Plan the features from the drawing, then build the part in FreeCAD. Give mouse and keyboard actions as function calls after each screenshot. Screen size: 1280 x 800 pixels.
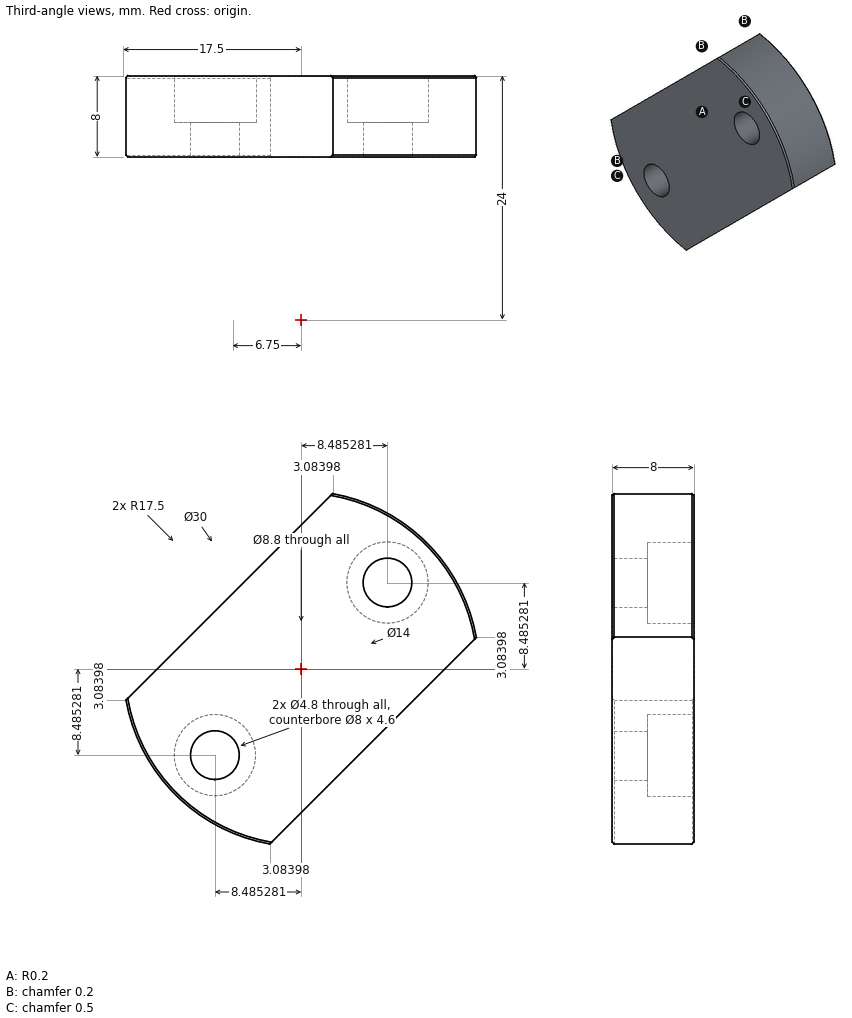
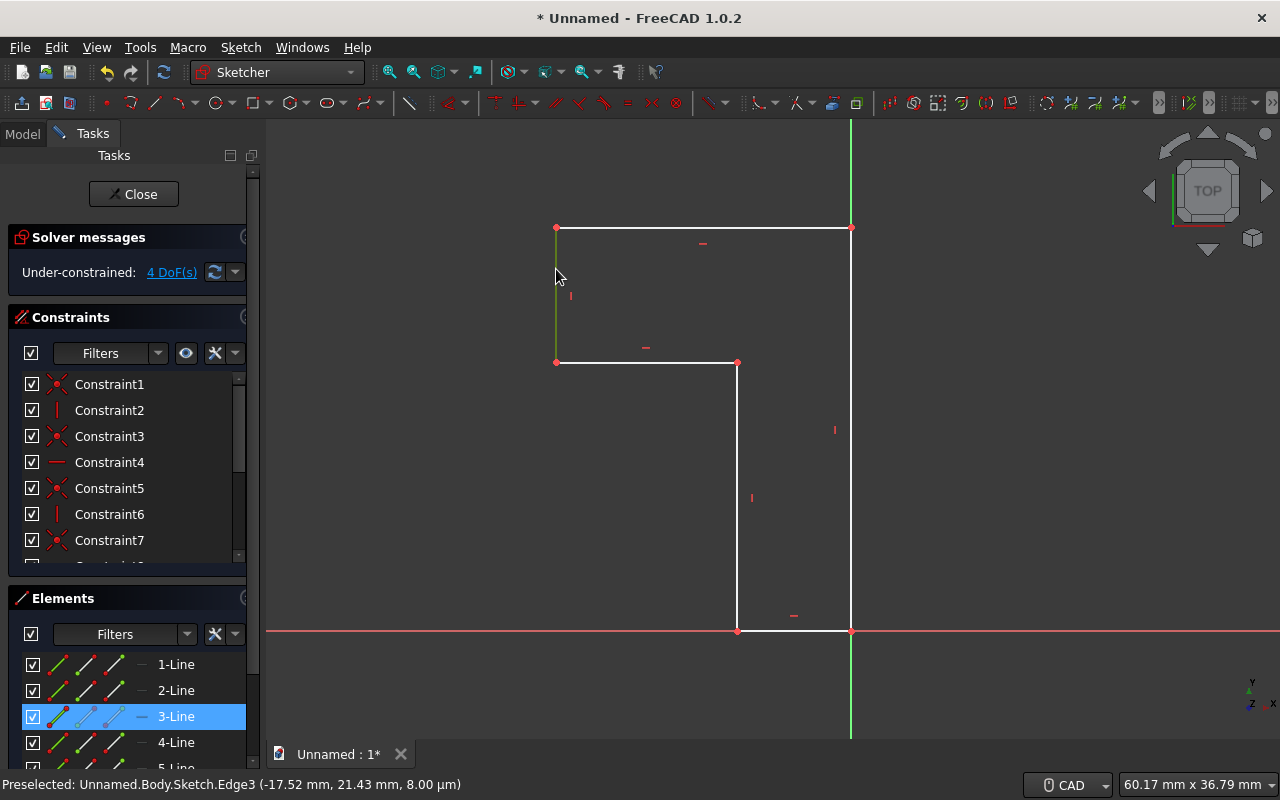
key(i)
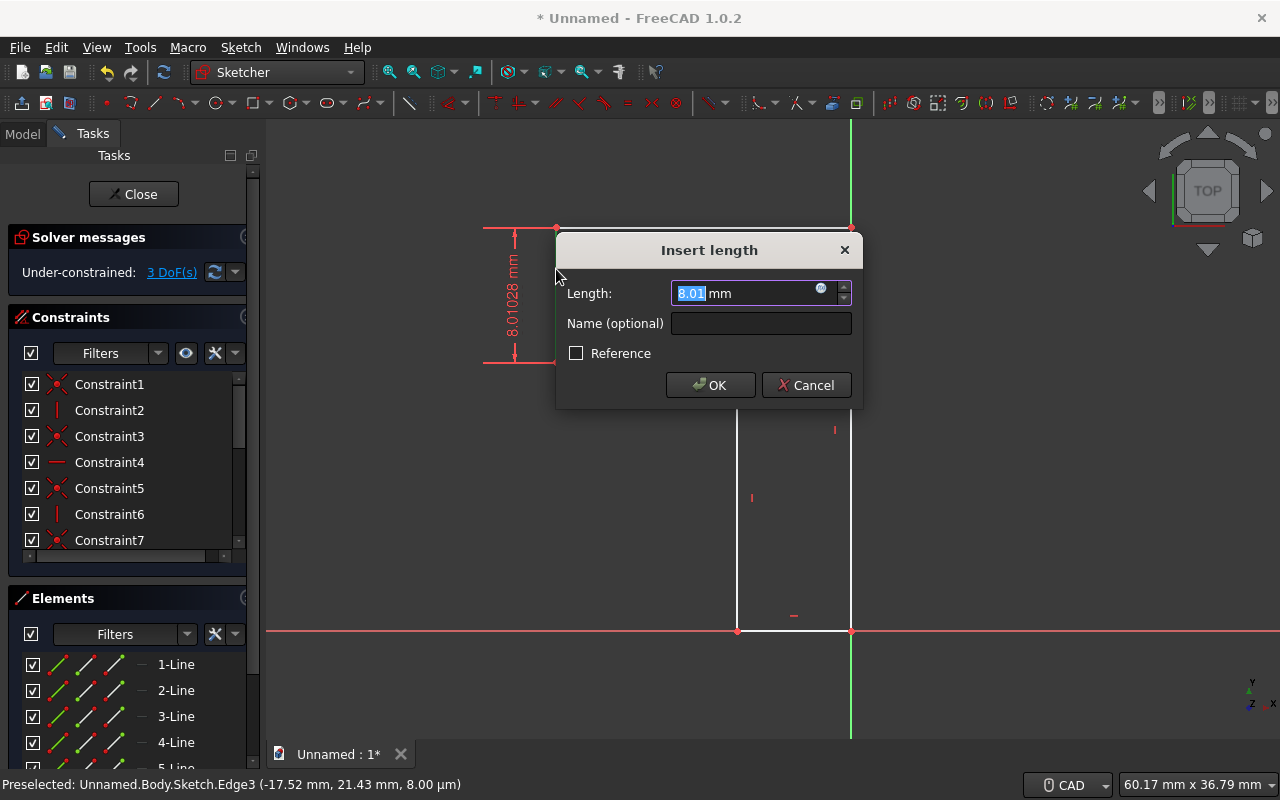
text(8)
key(Return)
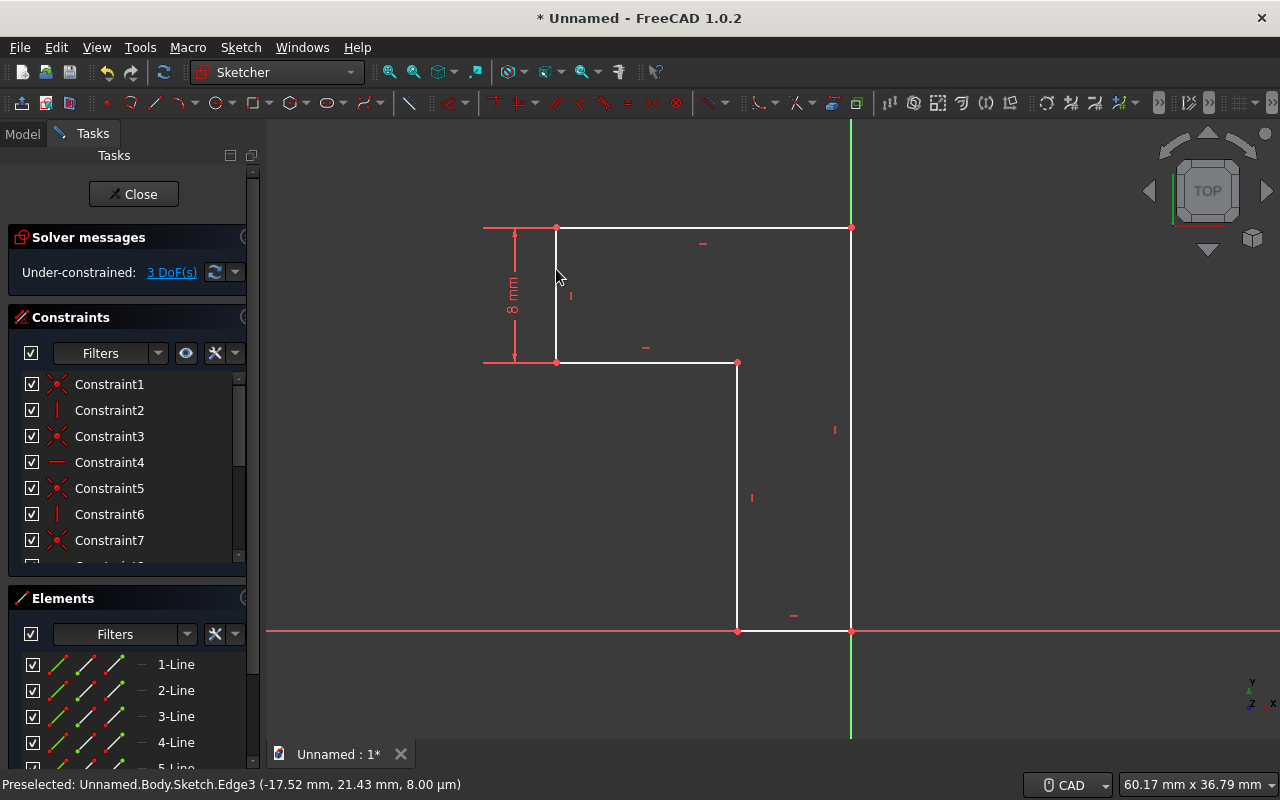
click(851, 510)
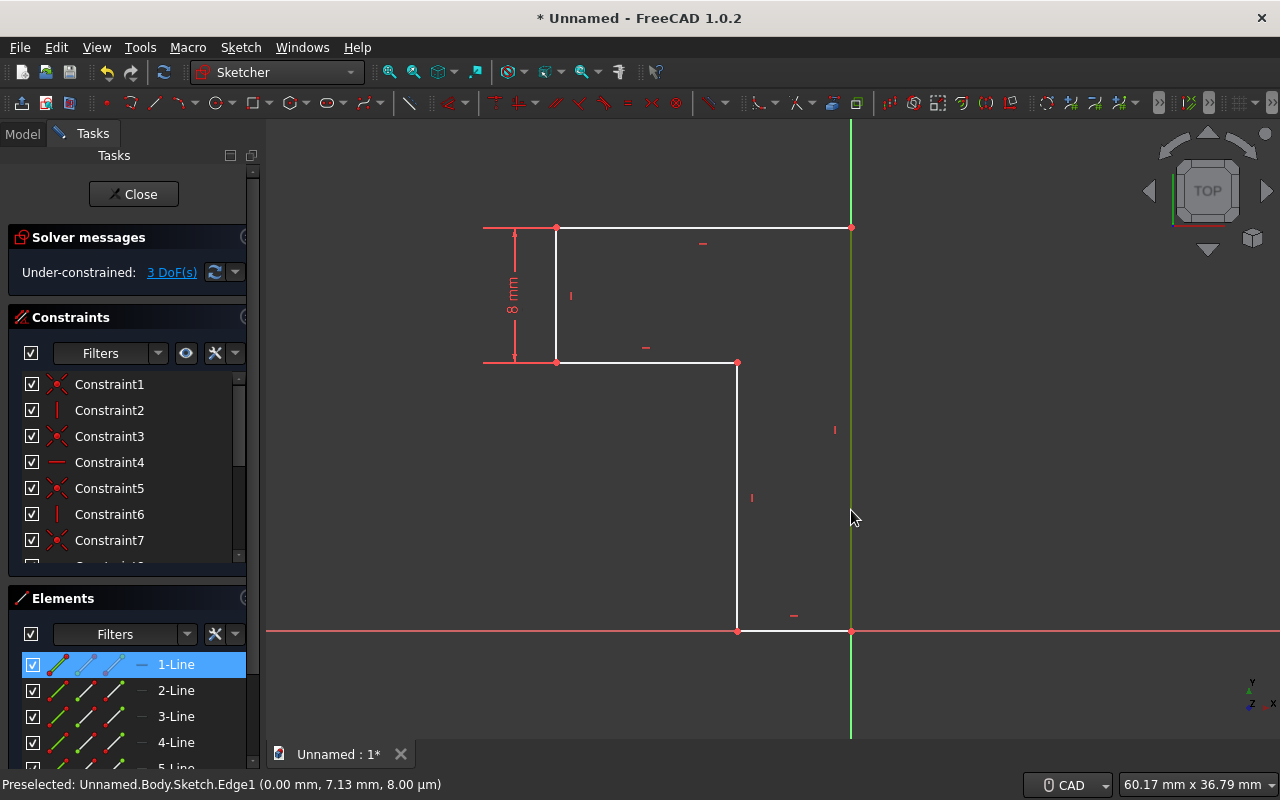
click(468, 104)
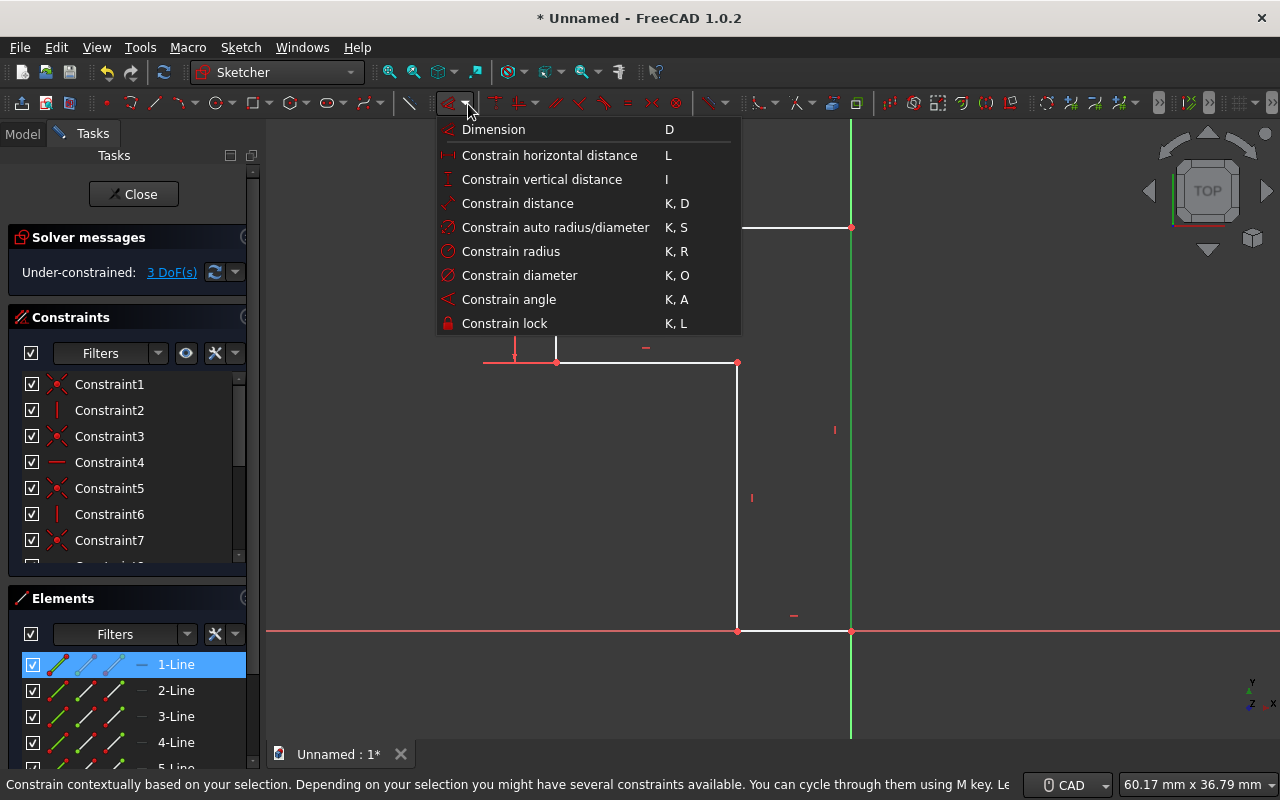
click(589, 179)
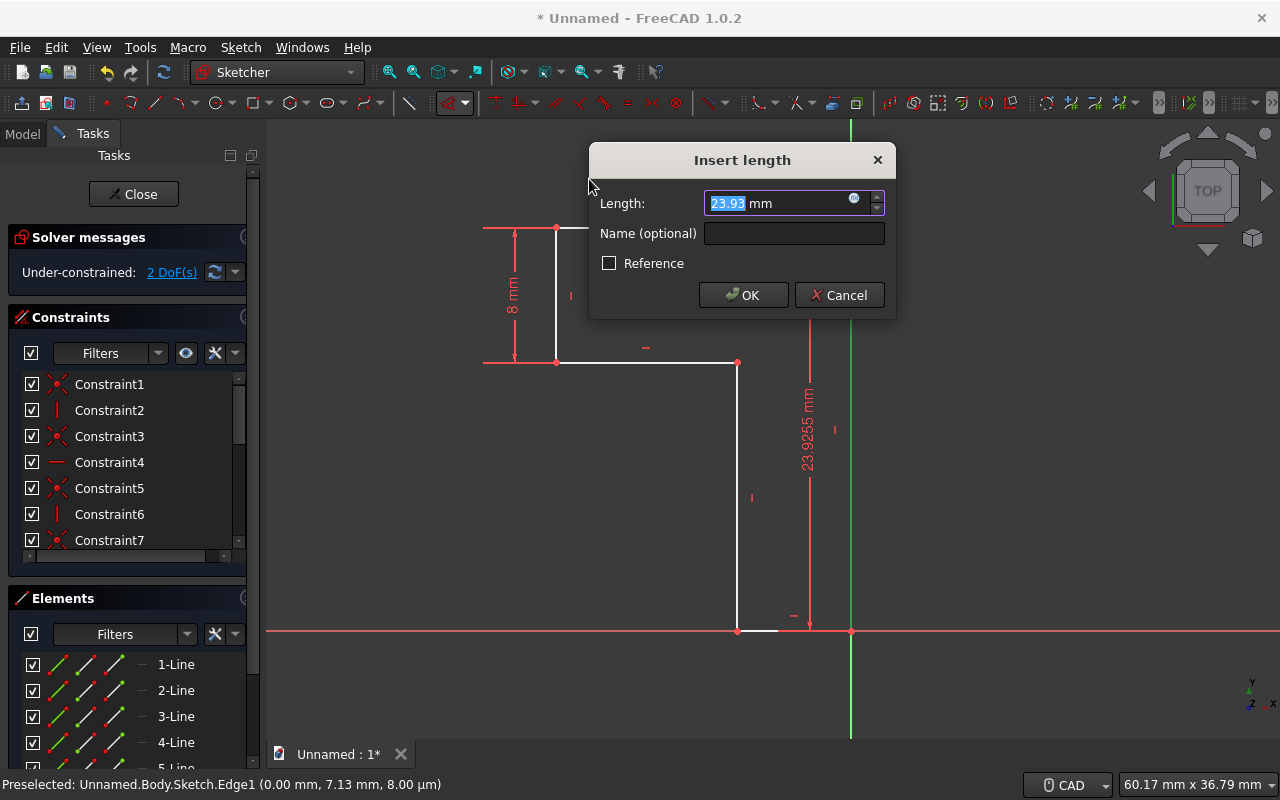
text(24)
key(Return)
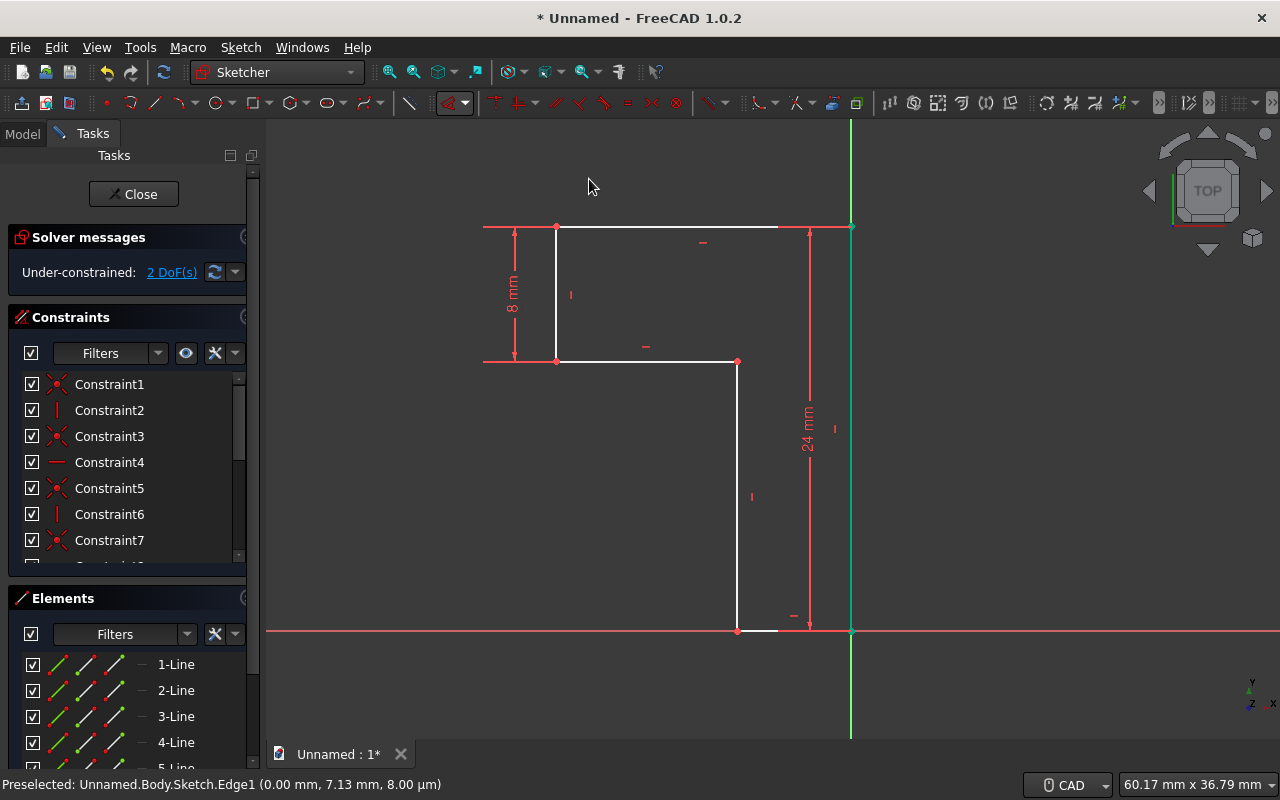
click(763, 227)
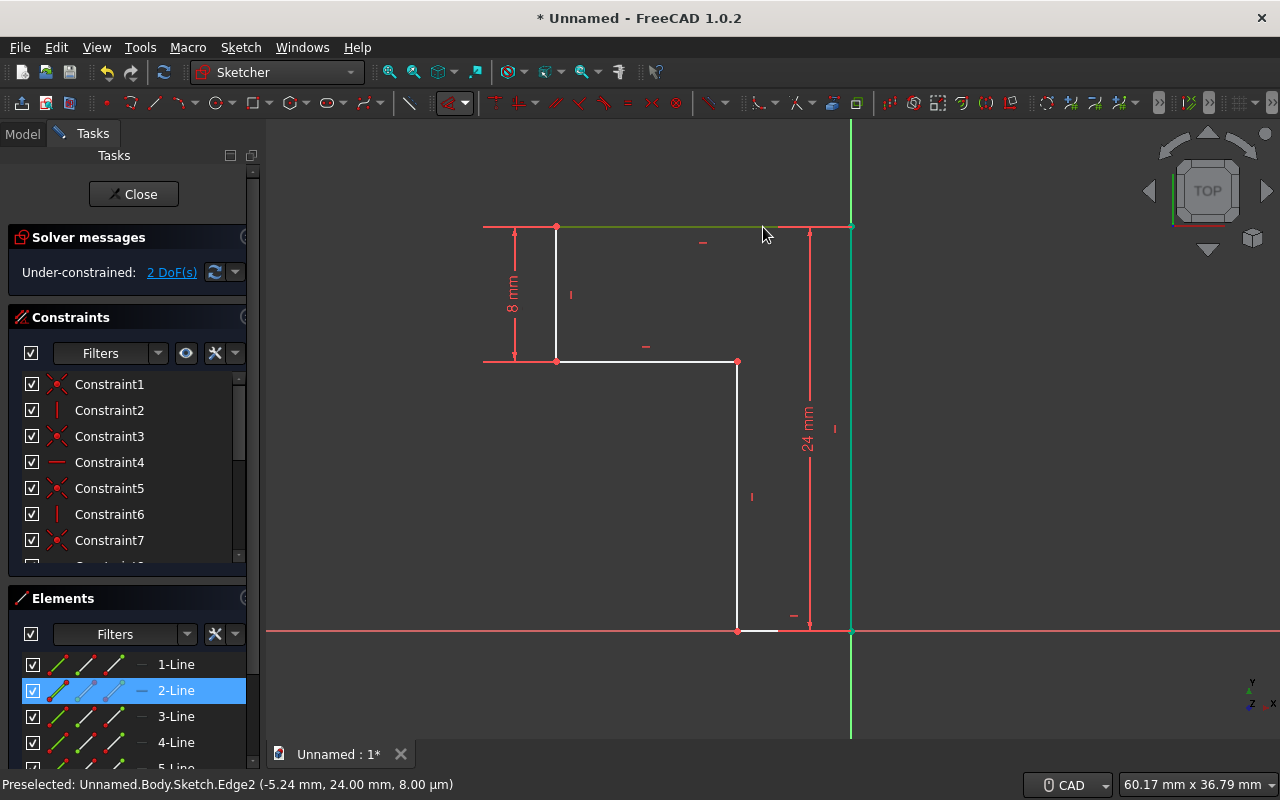
click(468, 104)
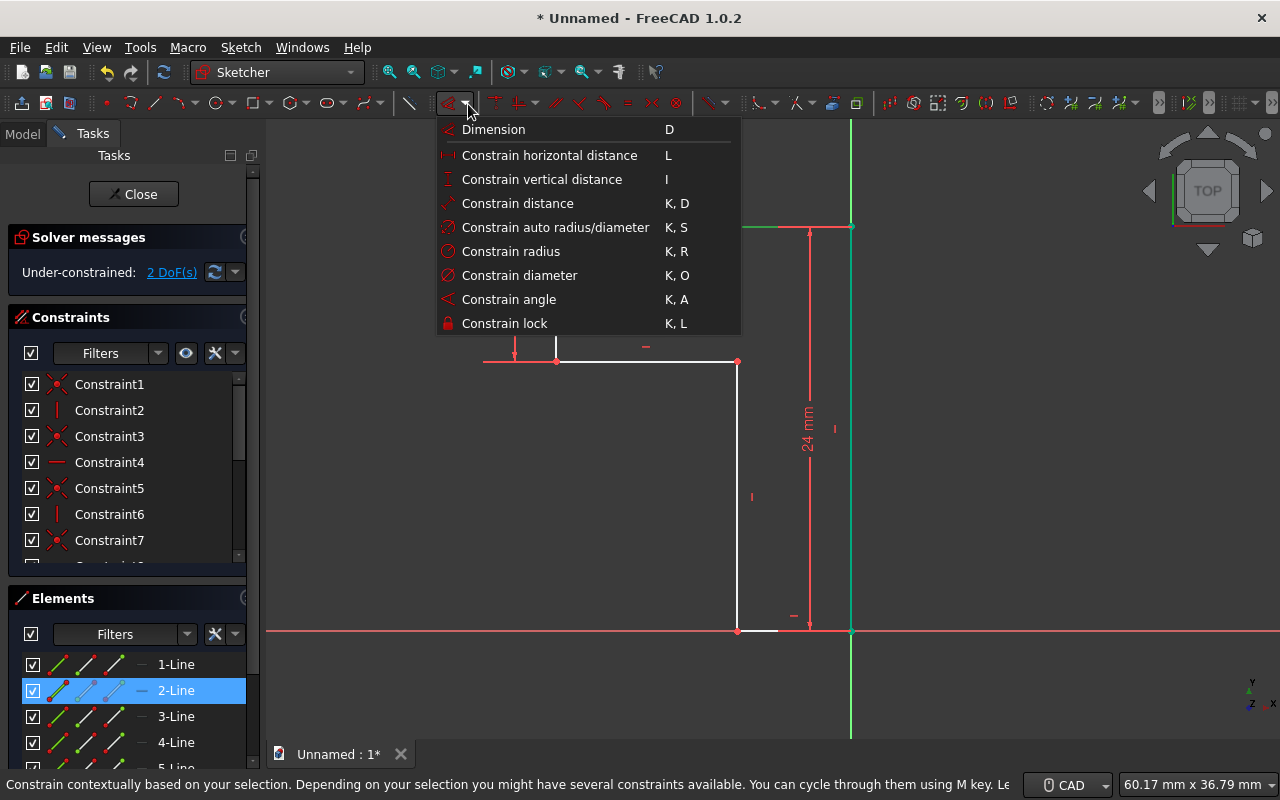
click(589, 155)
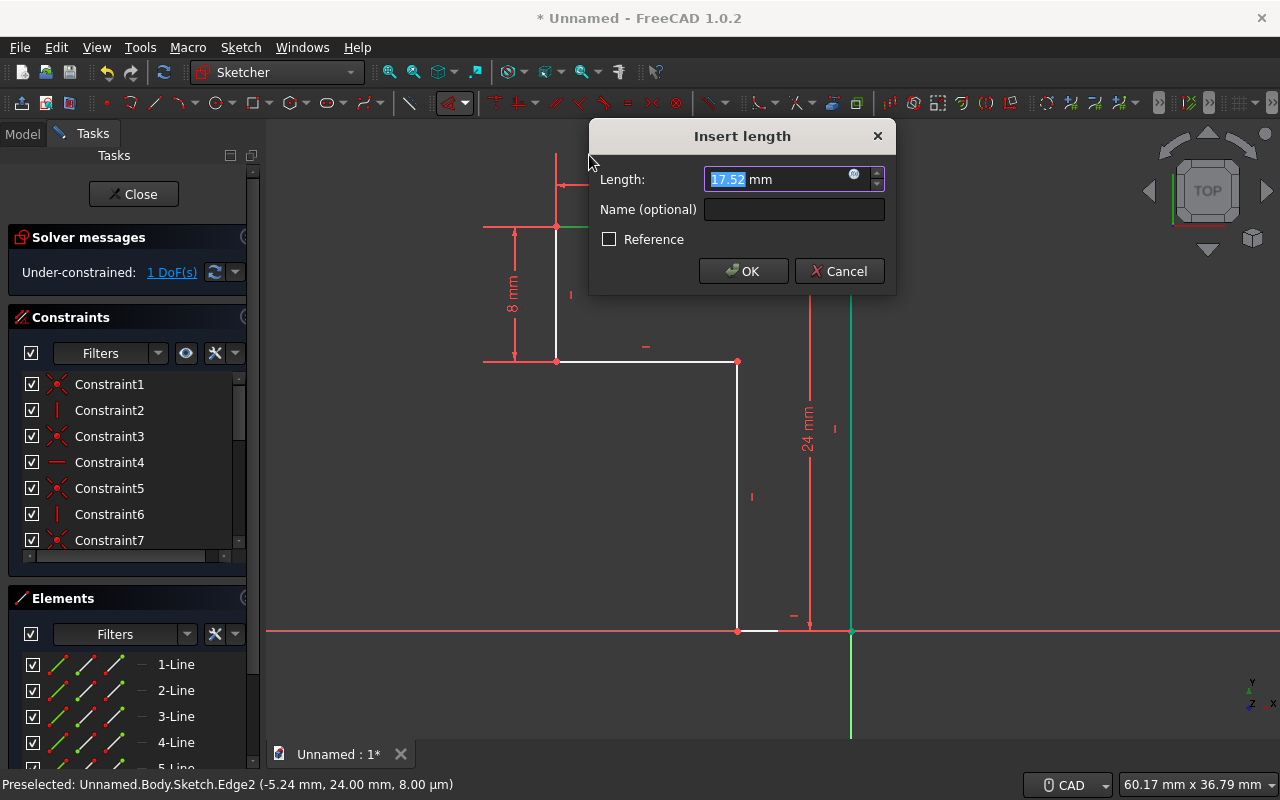
text(17.5)
key(Return)